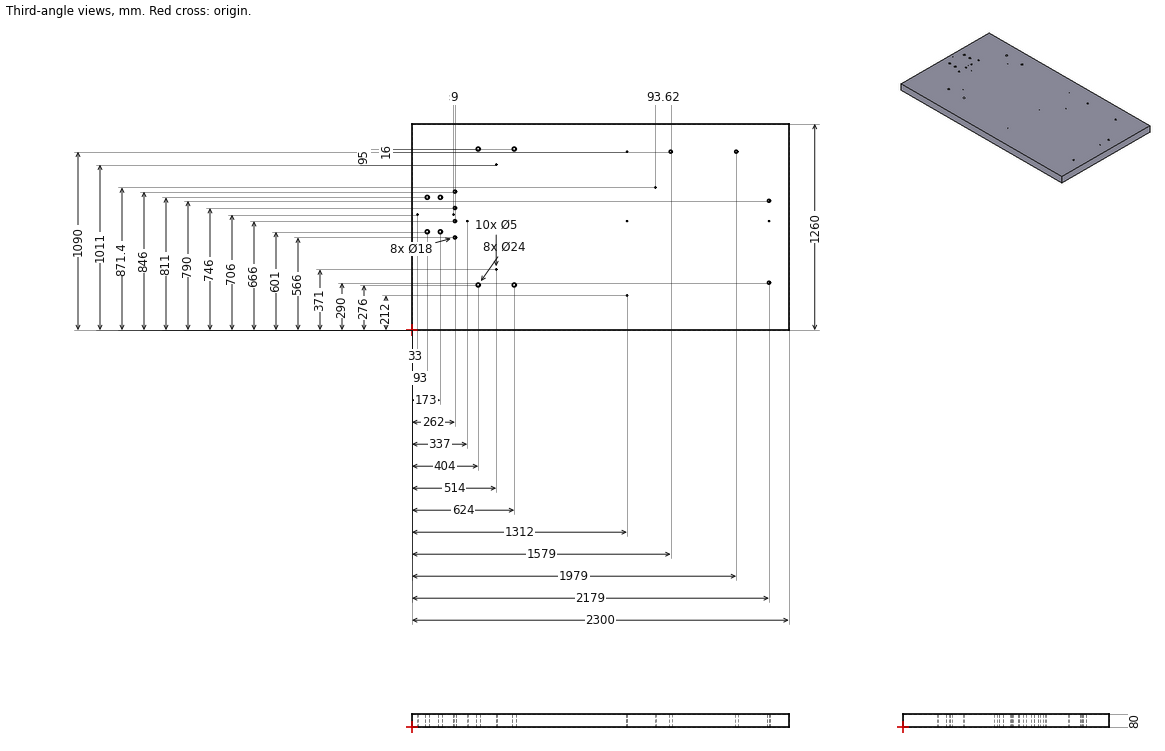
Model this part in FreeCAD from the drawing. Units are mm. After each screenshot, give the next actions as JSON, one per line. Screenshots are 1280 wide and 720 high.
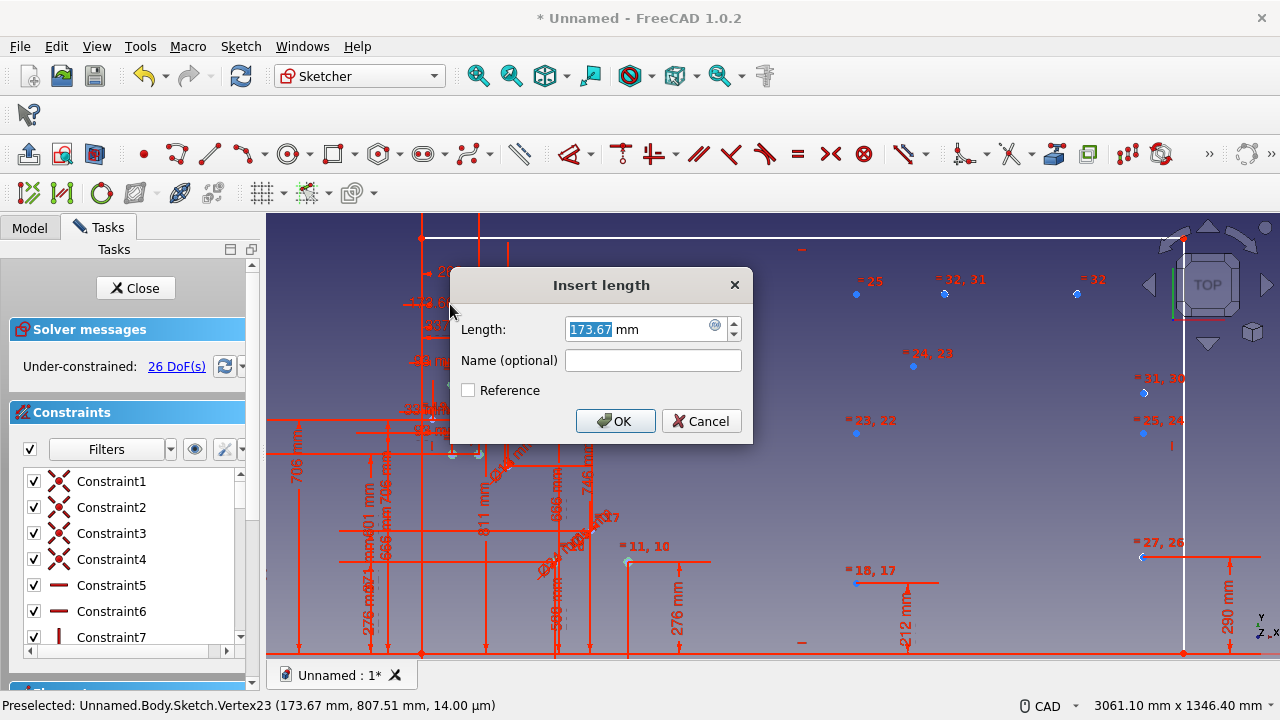
{"action": "type", "text": "173"}
{"action": "key", "text": "Return"}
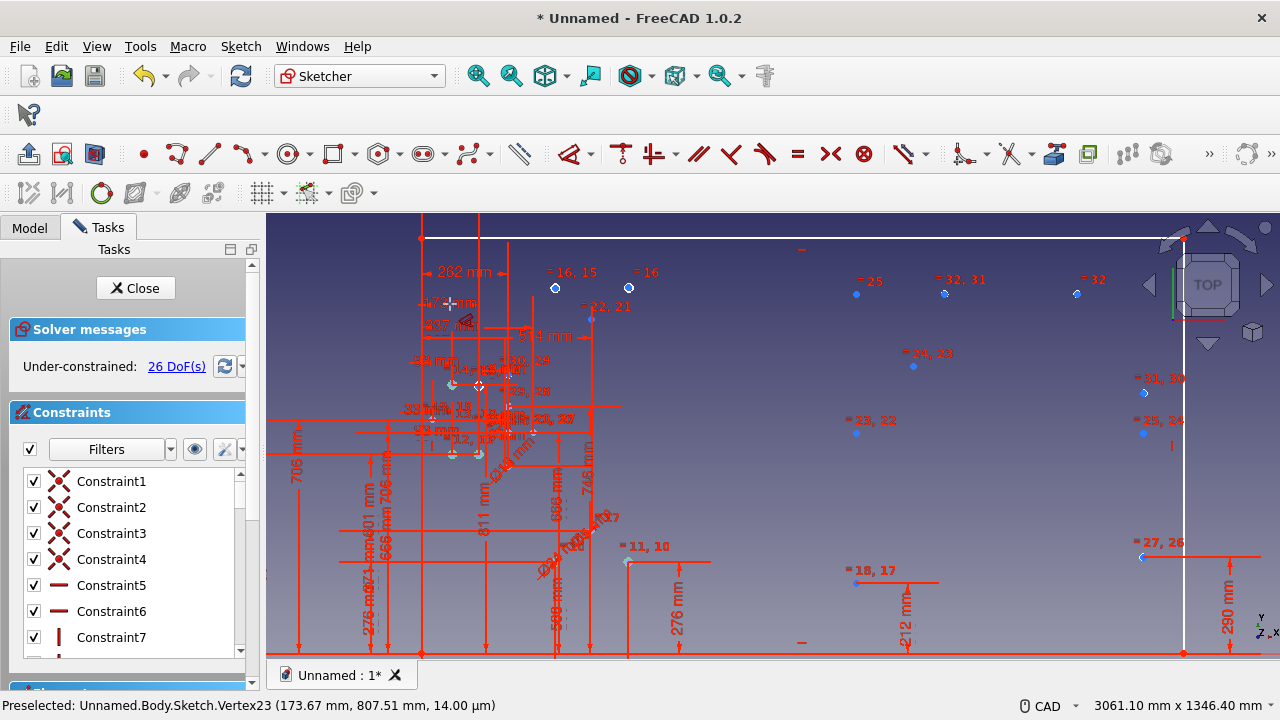
{"action": "left_click", "coordinate": [479, 386]}
{"action": "left_click", "coordinate": [340, 423]}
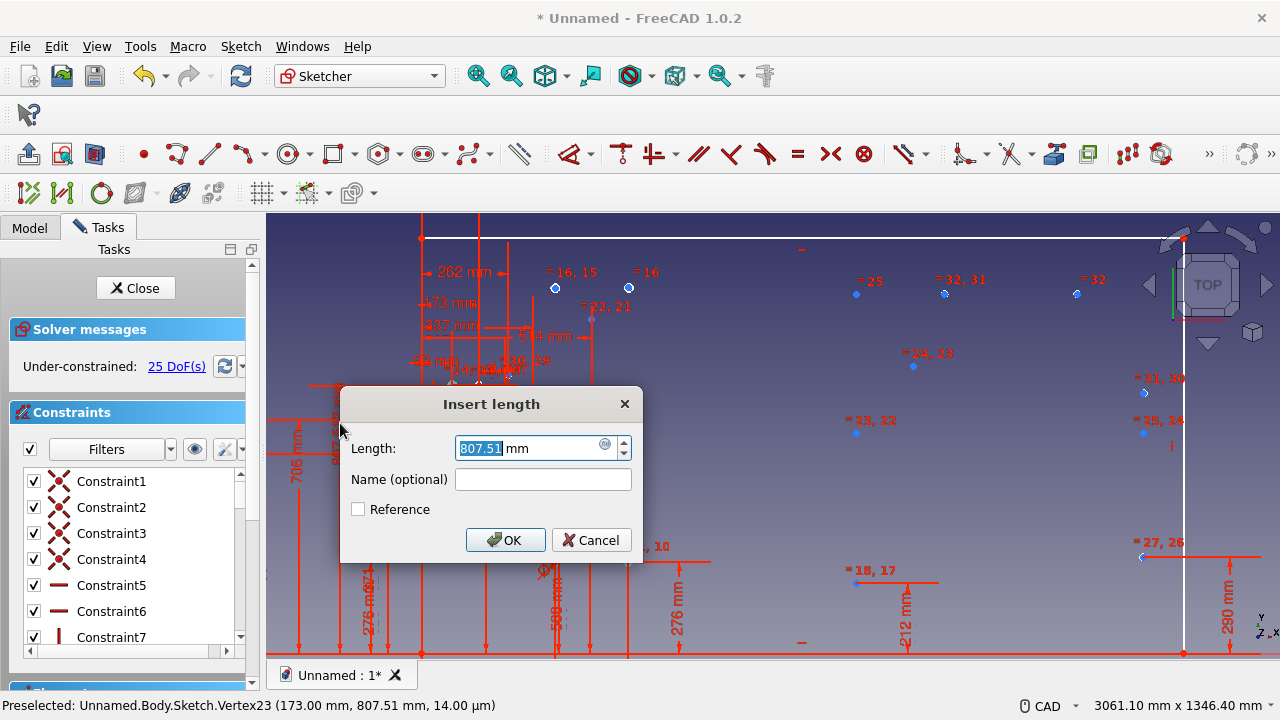
{"action": "type", "text": "811"}
{"action": "key", "text": "Return"}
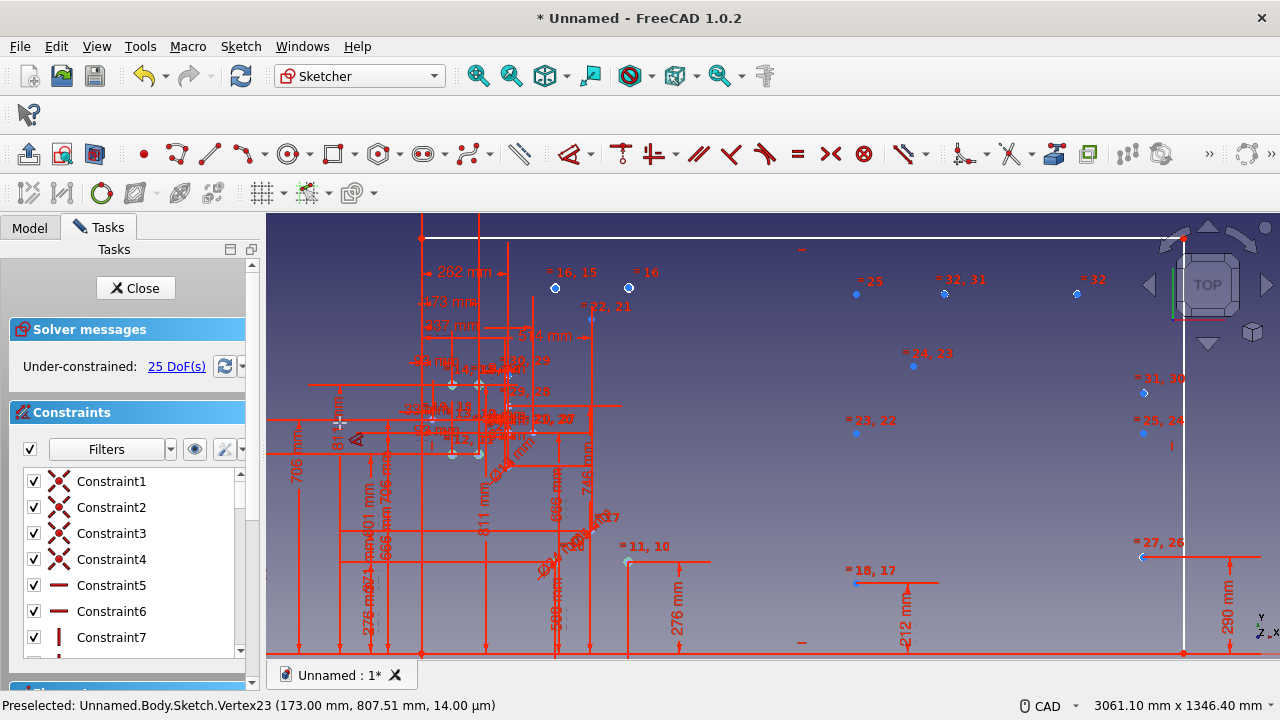
{"action": "left_click", "coordinate": [508, 375]}
{"action": "left_click", "coordinate": [590, 444]}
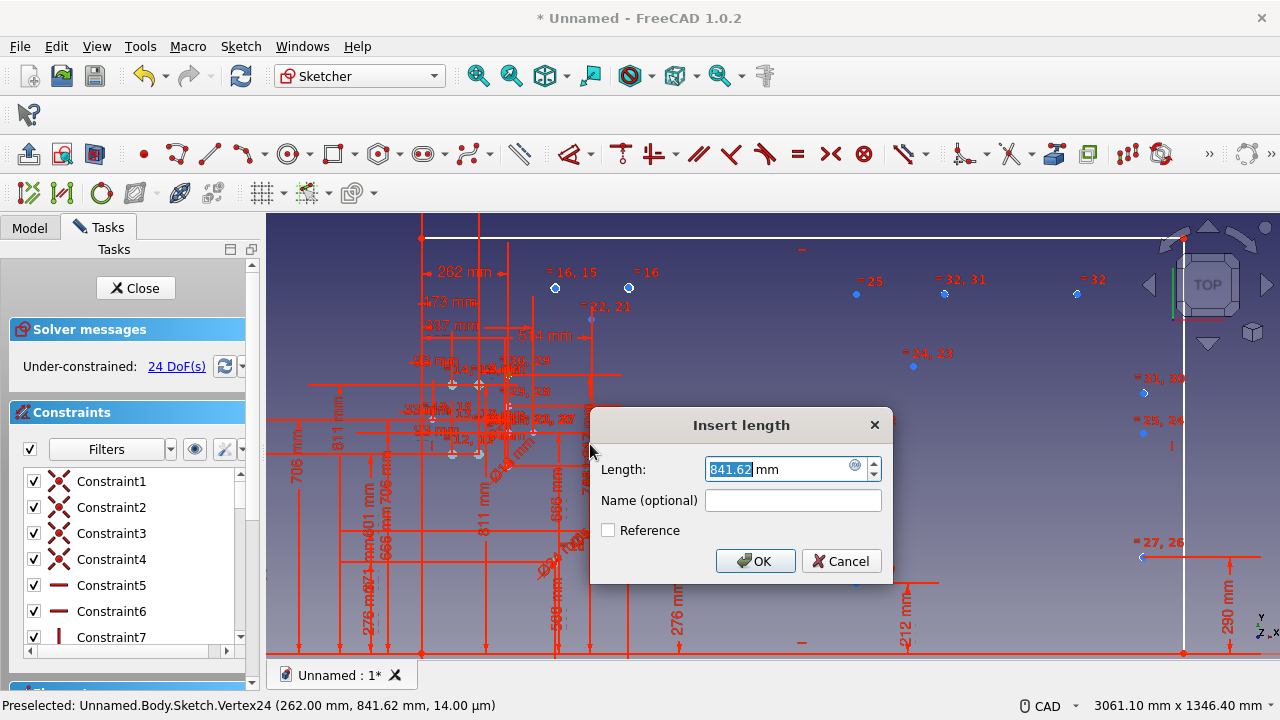
{"action": "type", "text": "846"}
{"action": "key", "text": "Return"}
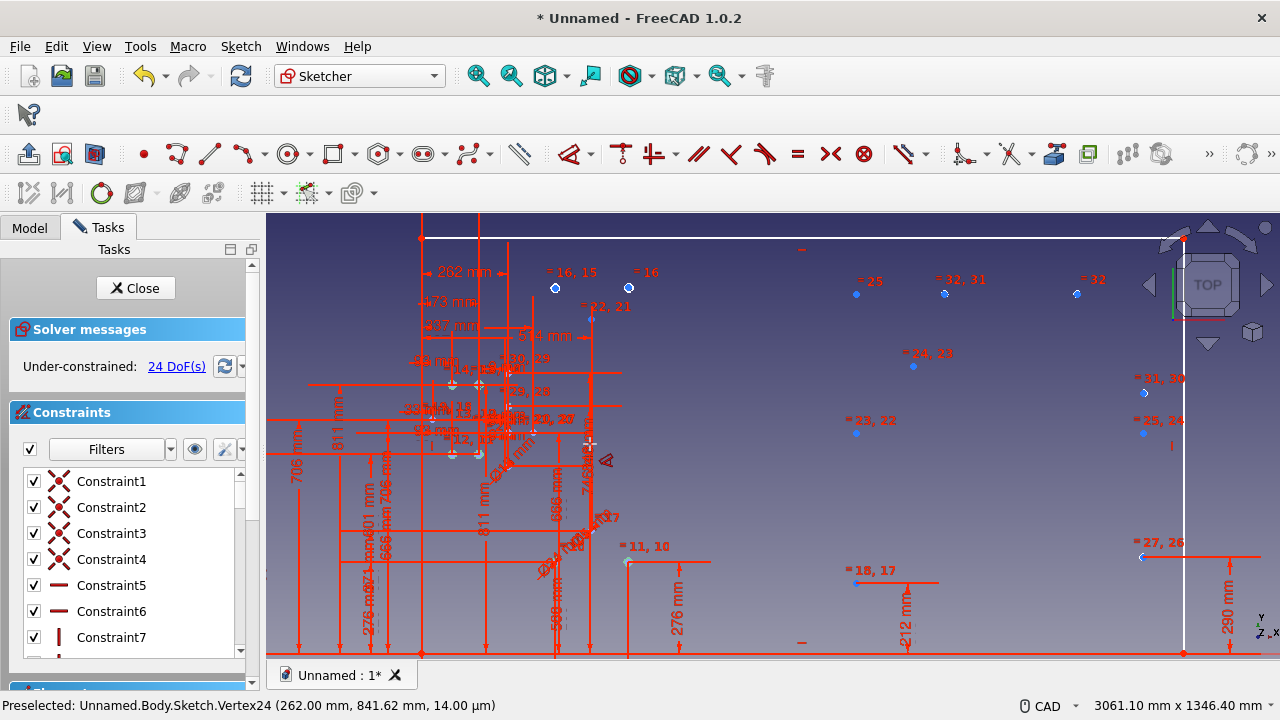
{"action": "left_click", "coordinate": [591, 320]}
{"action": "left_click", "coordinate": [545, 262]}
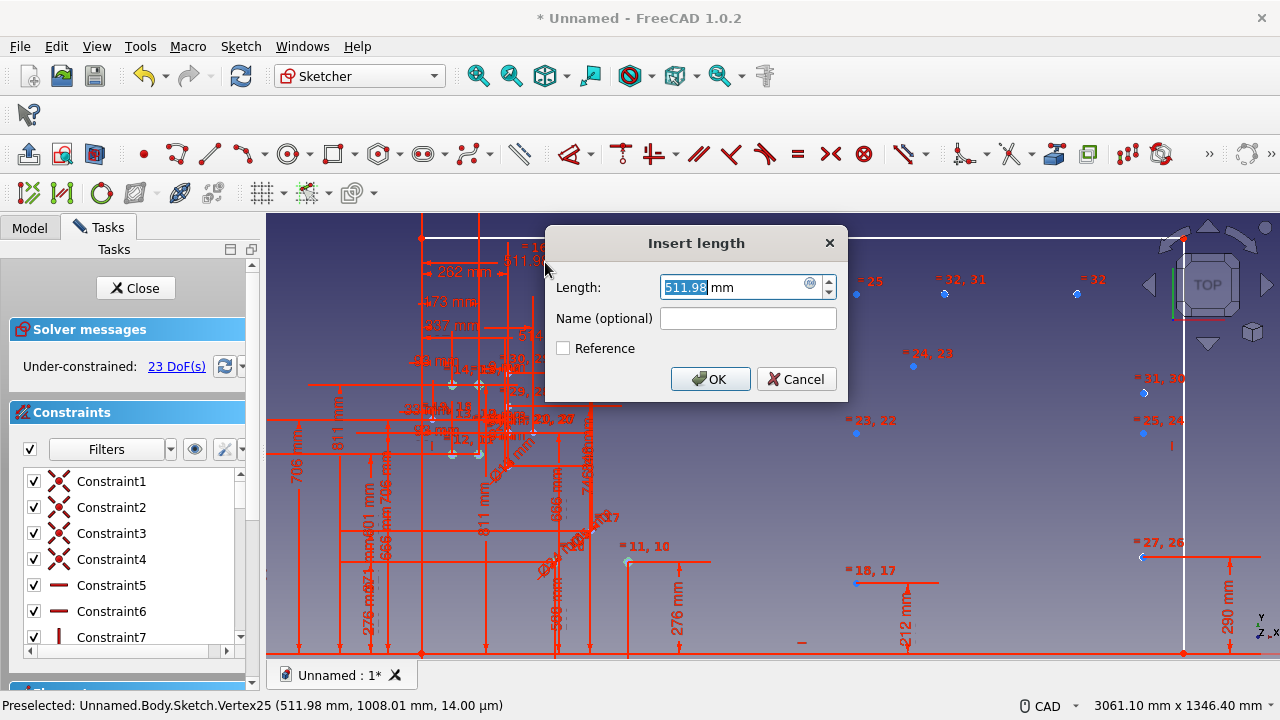
{"action": "type", "text": "514"}
{"action": "key", "text": "Return"}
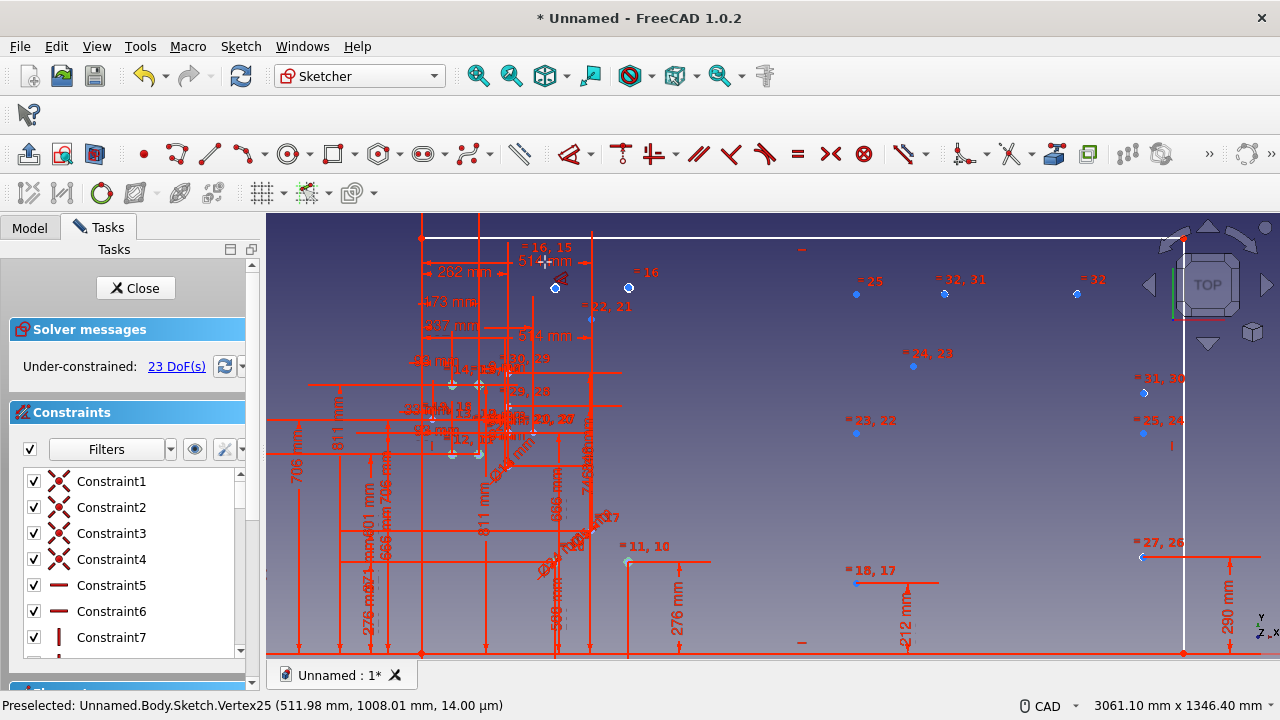
{"action": "left_click", "coordinate": [555, 288]}
{"action": "left_click", "coordinate": [488, 254]}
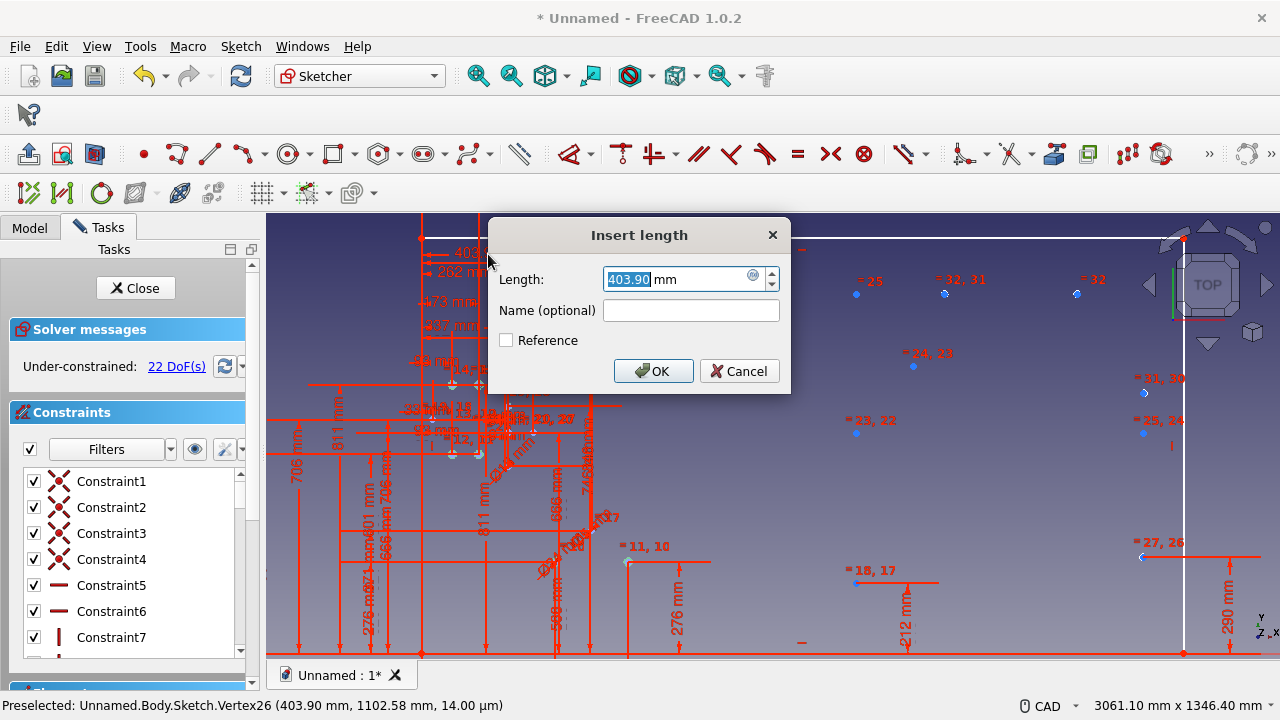
{"action": "type", "text": "404"}
{"action": "key", "text": "Return"}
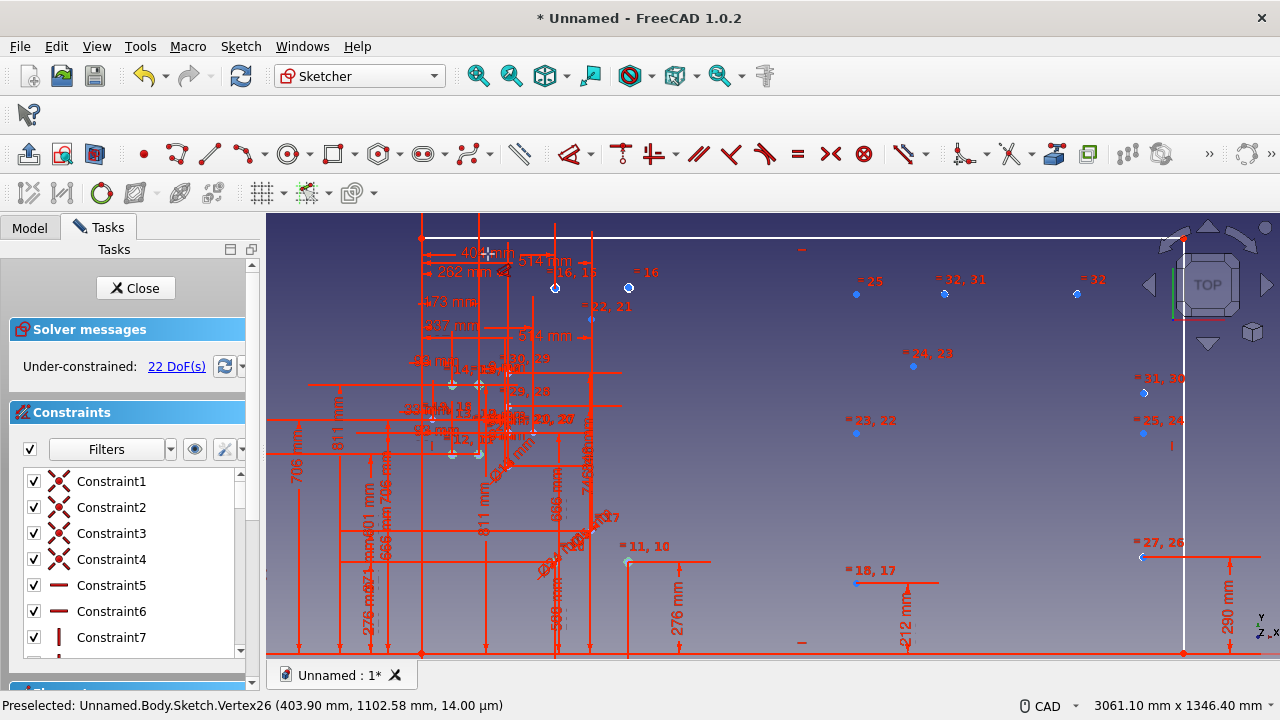
{"action": "left_click", "coordinate": [629, 288]}
{"action": "left_click", "coordinate": [453, 254]}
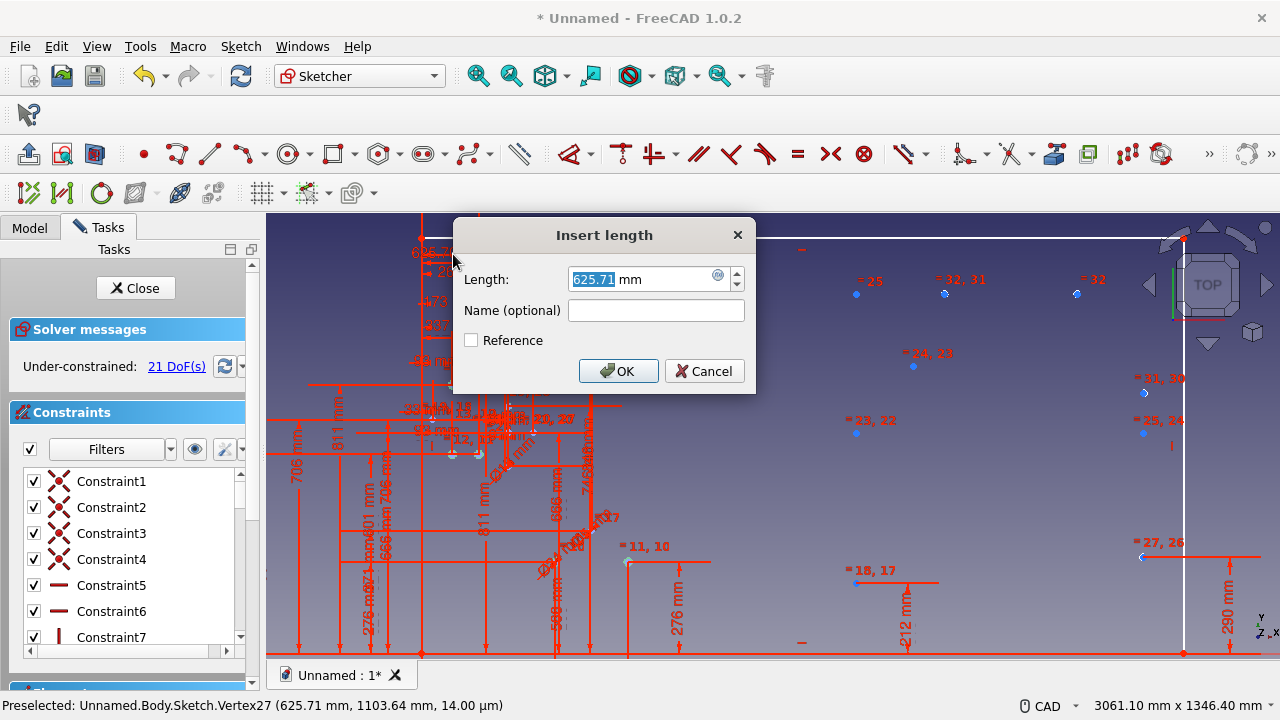
{"action": "type", "text": "624"}
{"action": "key", "text": "Return"}